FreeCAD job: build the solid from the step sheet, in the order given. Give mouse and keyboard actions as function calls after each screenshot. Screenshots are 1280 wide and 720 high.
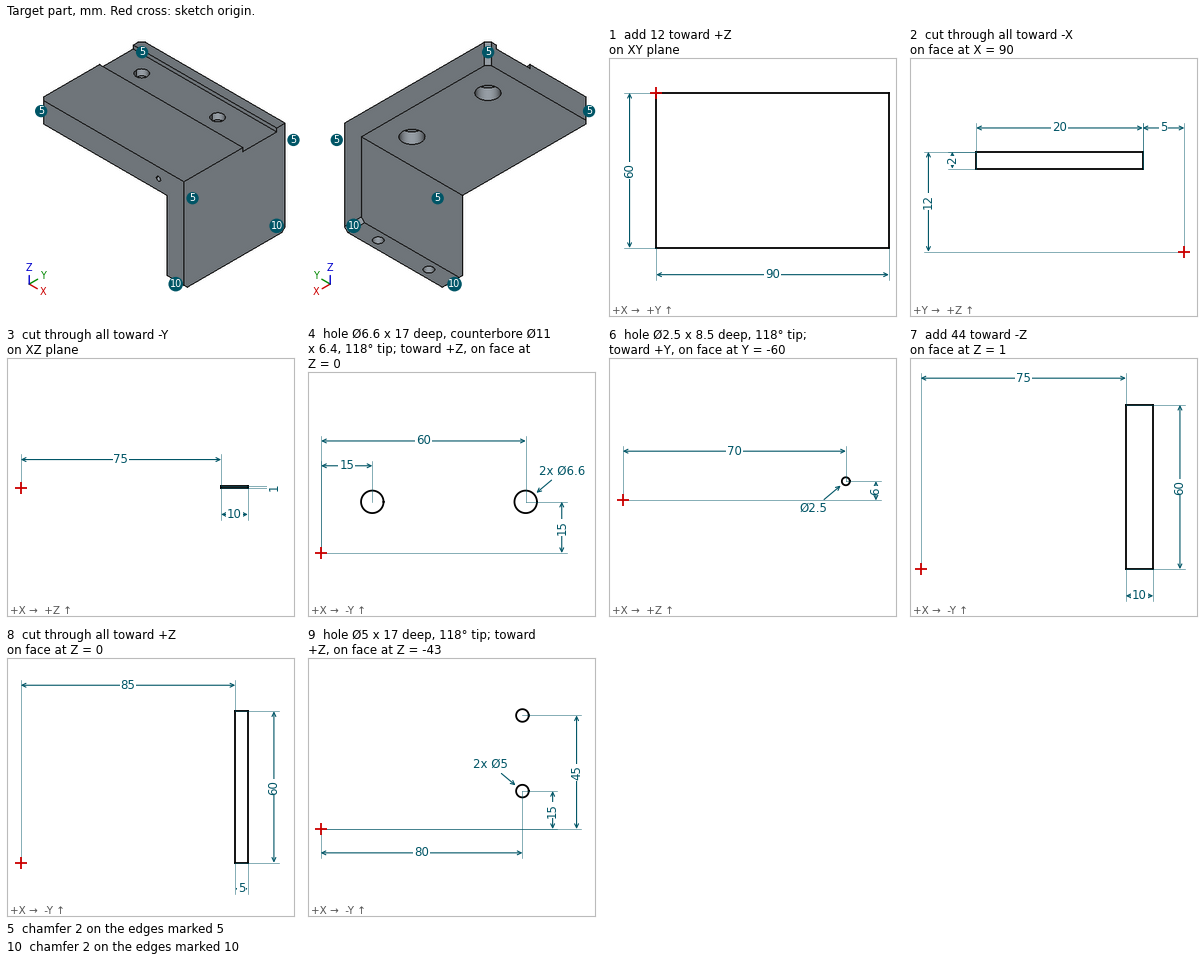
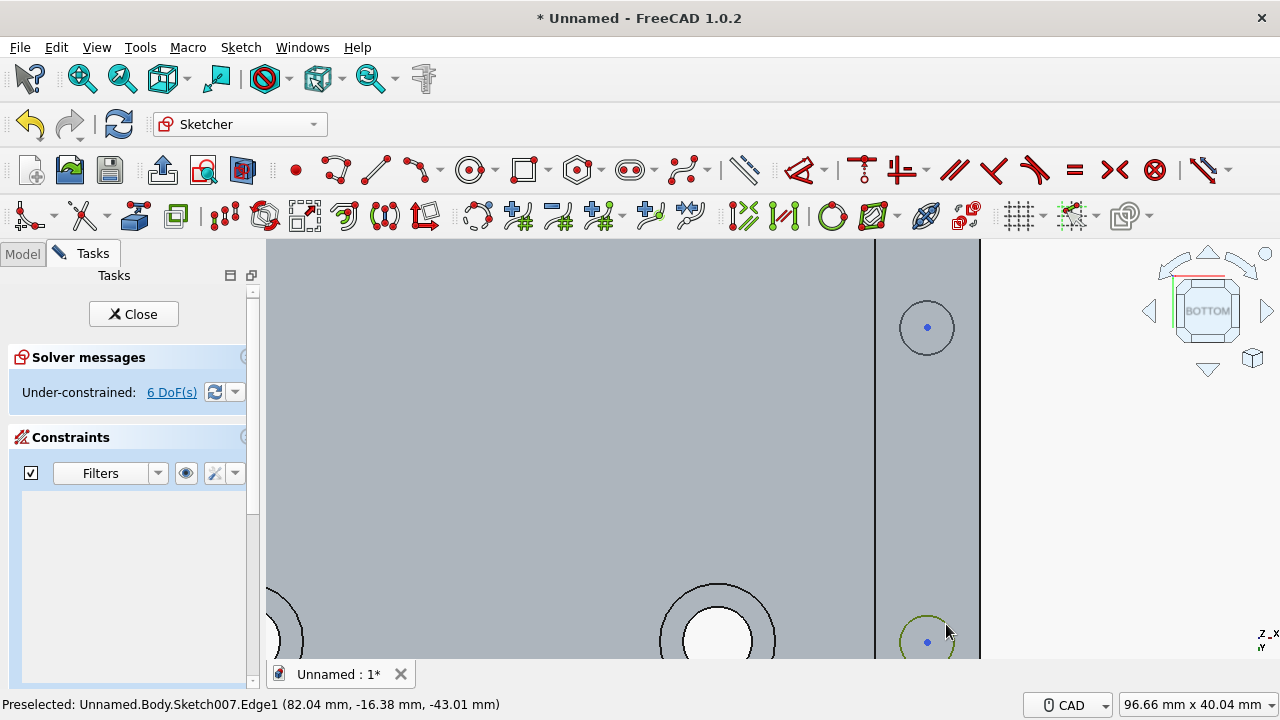
click(946, 309)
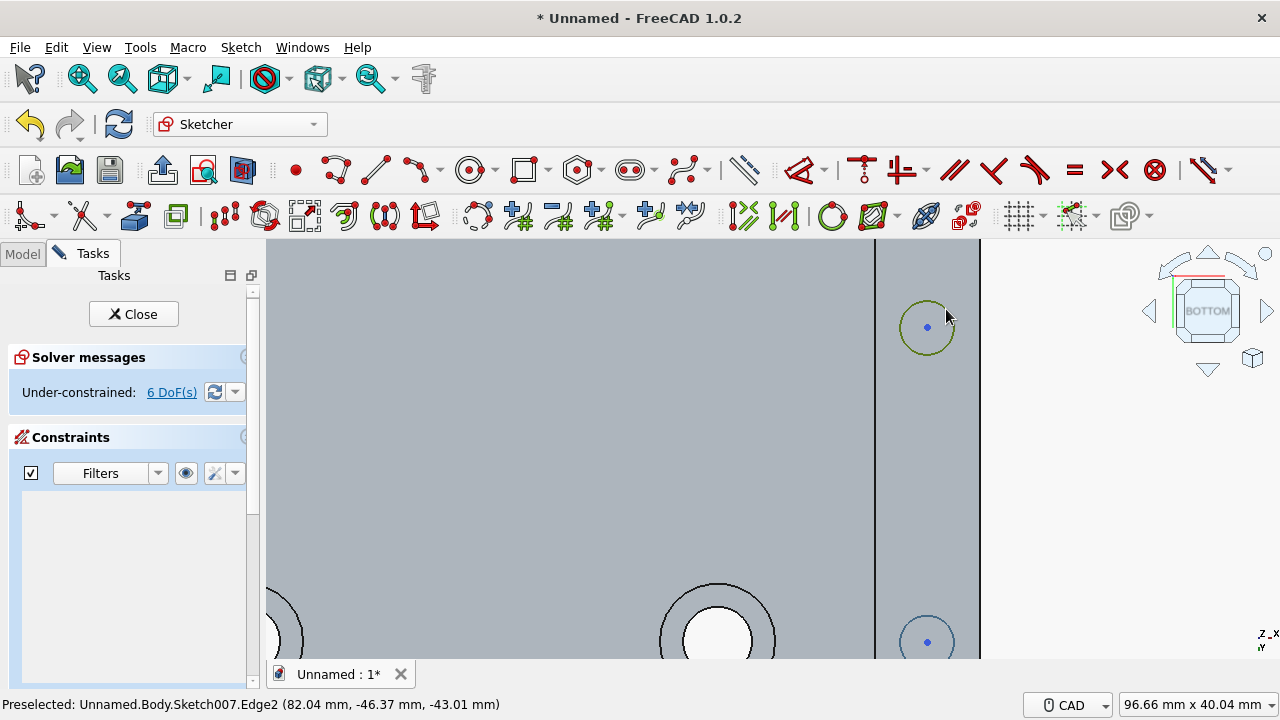
click(1076, 170)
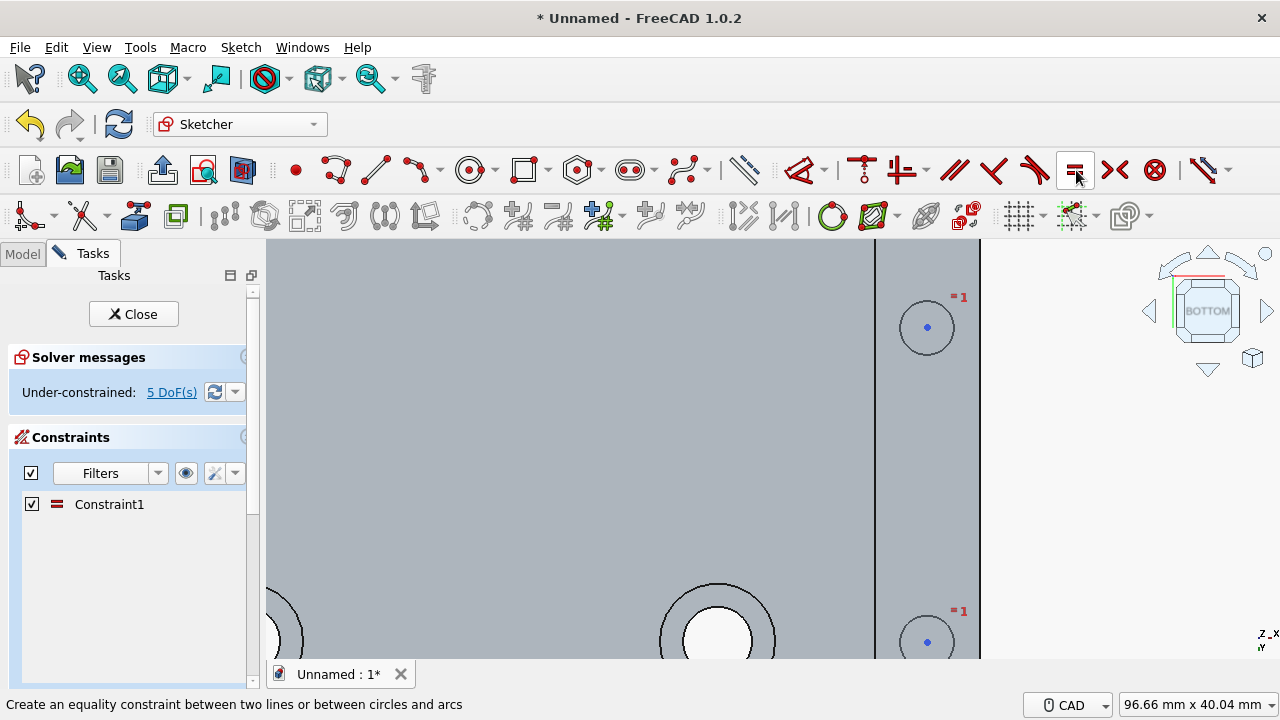
scroll(928, 327, down, 3)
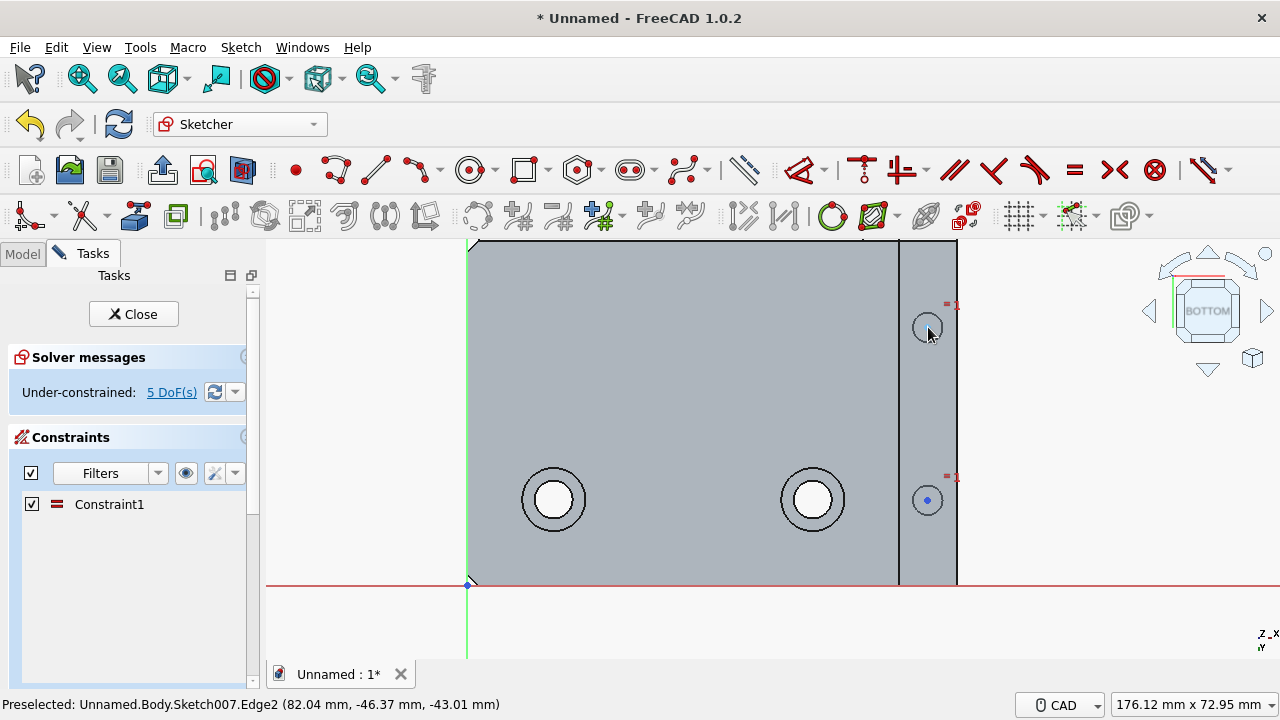
click(928, 500)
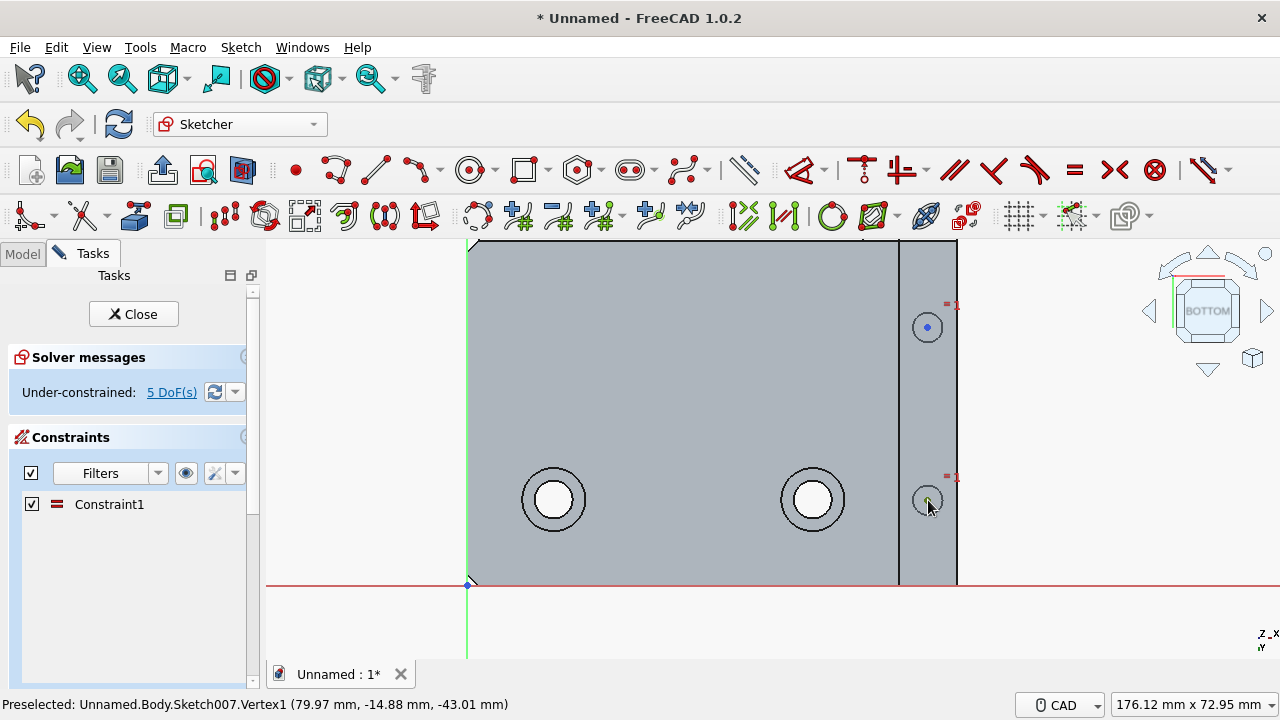
click(928, 328)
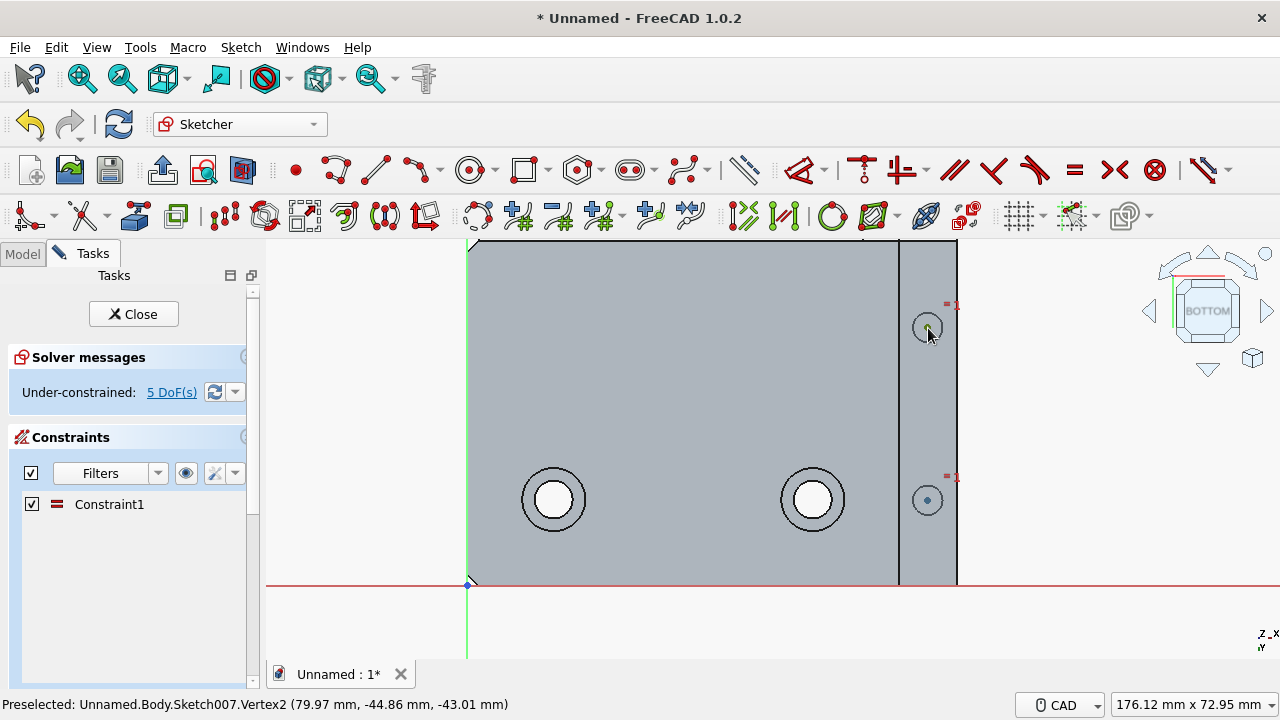
key(v)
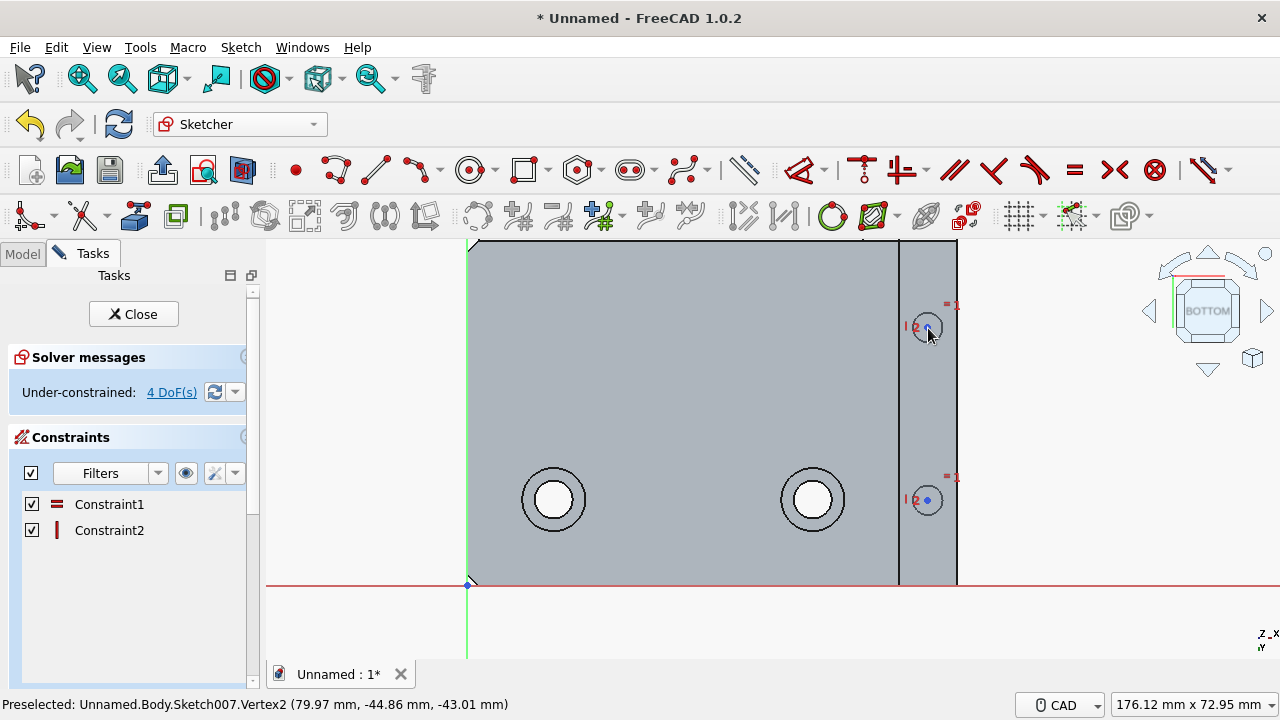
click(800, 170)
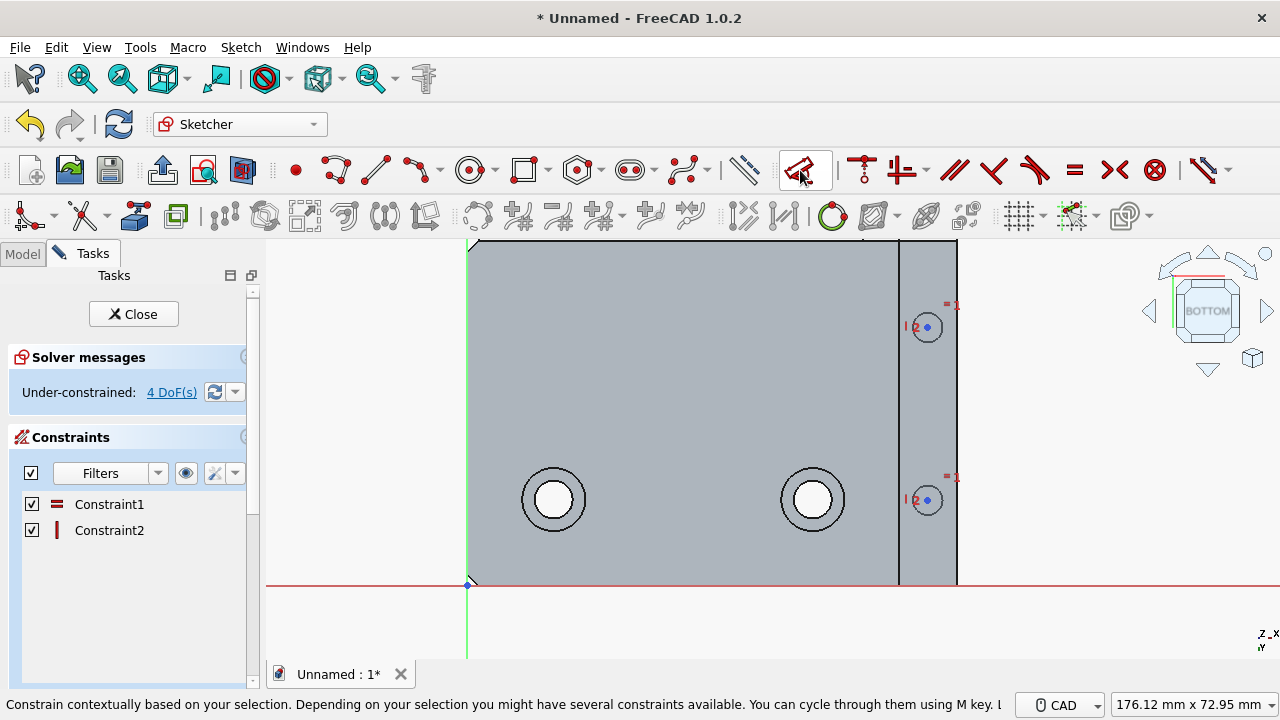
scroll(938, 490, up, 2)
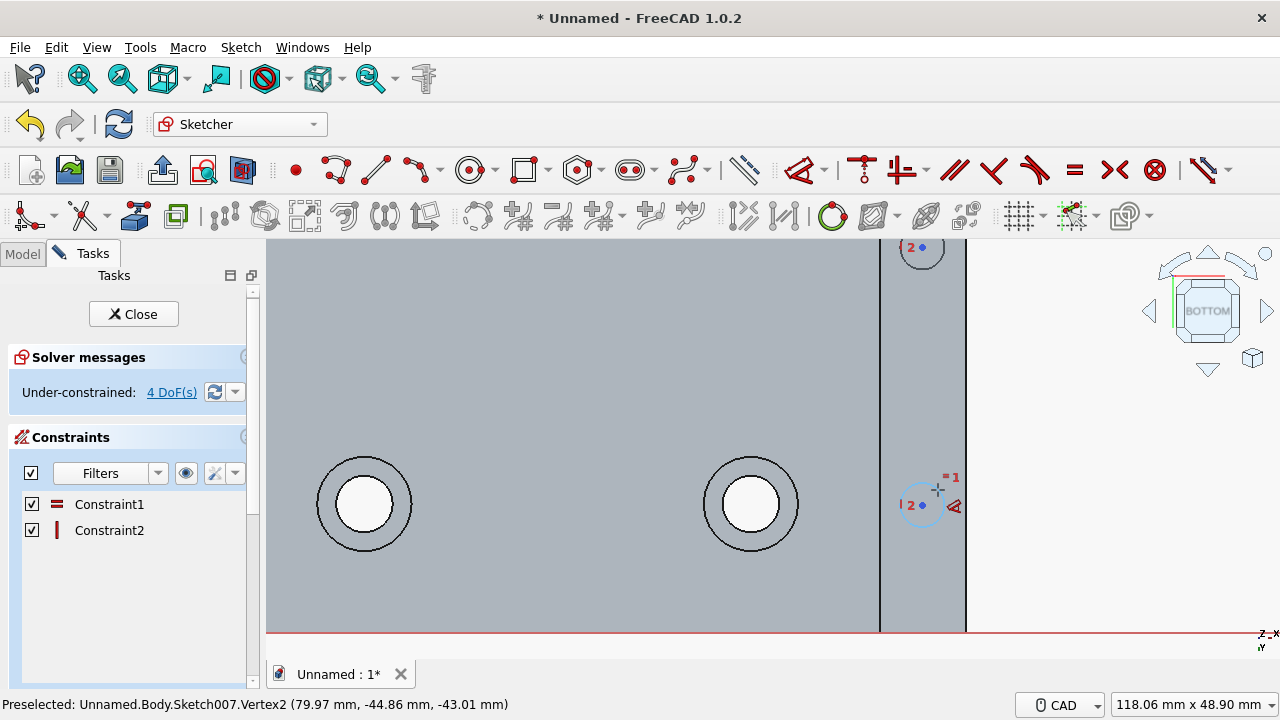
click(938, 489)
click(960, 466)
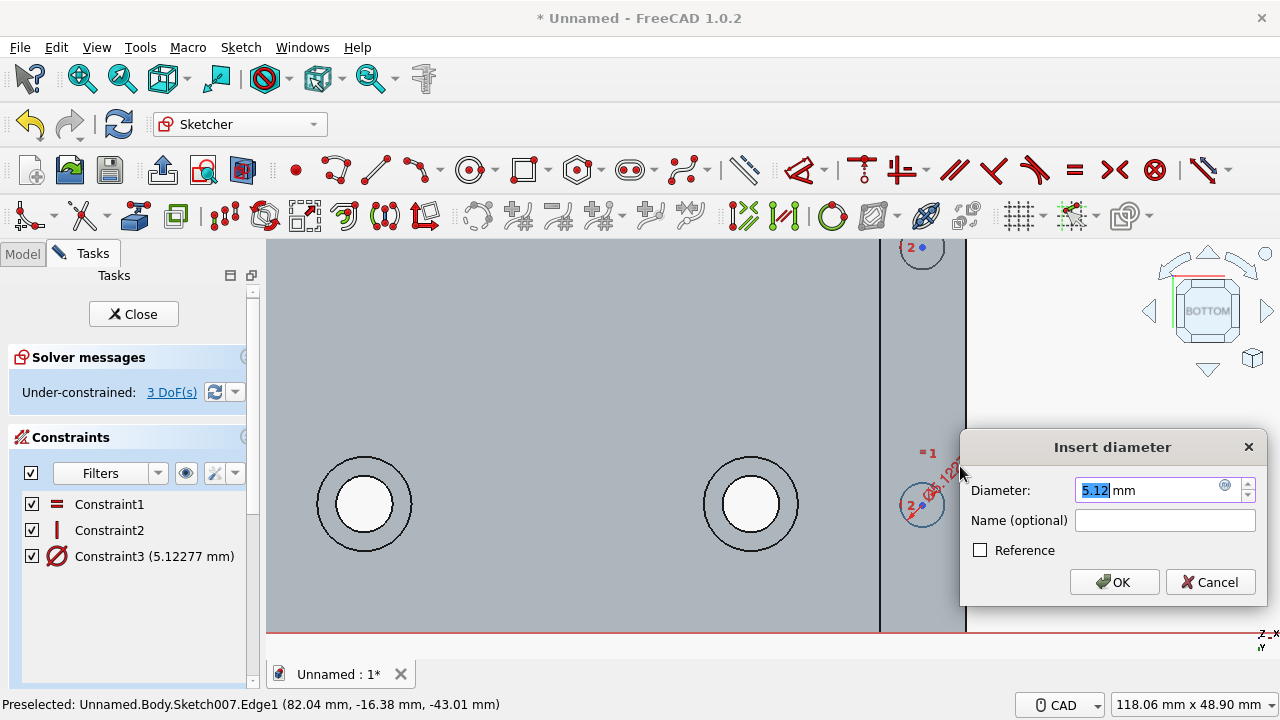
text(5)
key(Return)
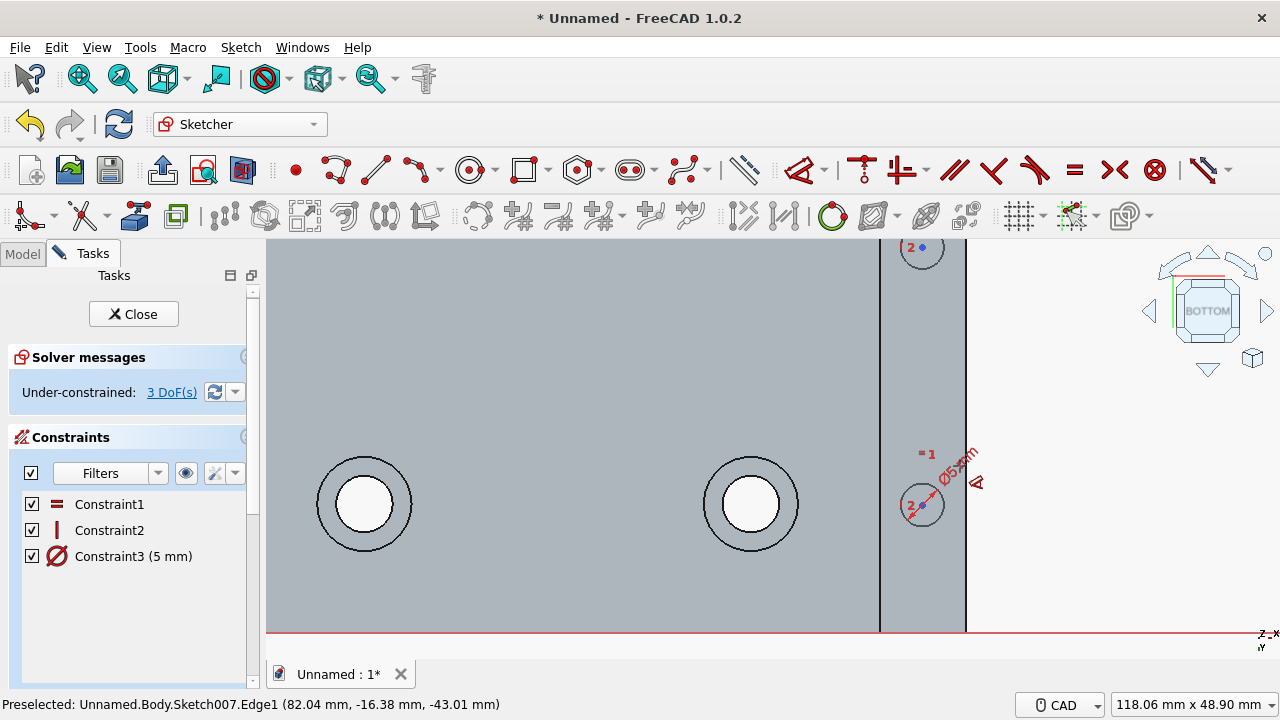
click(922, 505)
click(608, 471)